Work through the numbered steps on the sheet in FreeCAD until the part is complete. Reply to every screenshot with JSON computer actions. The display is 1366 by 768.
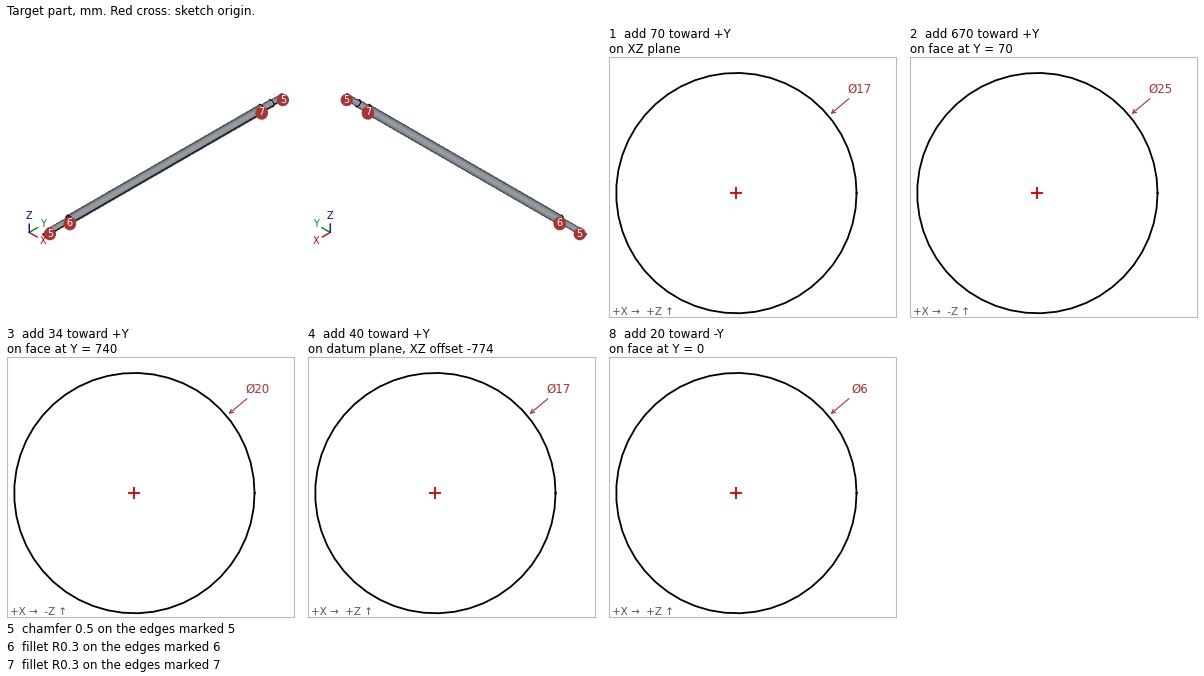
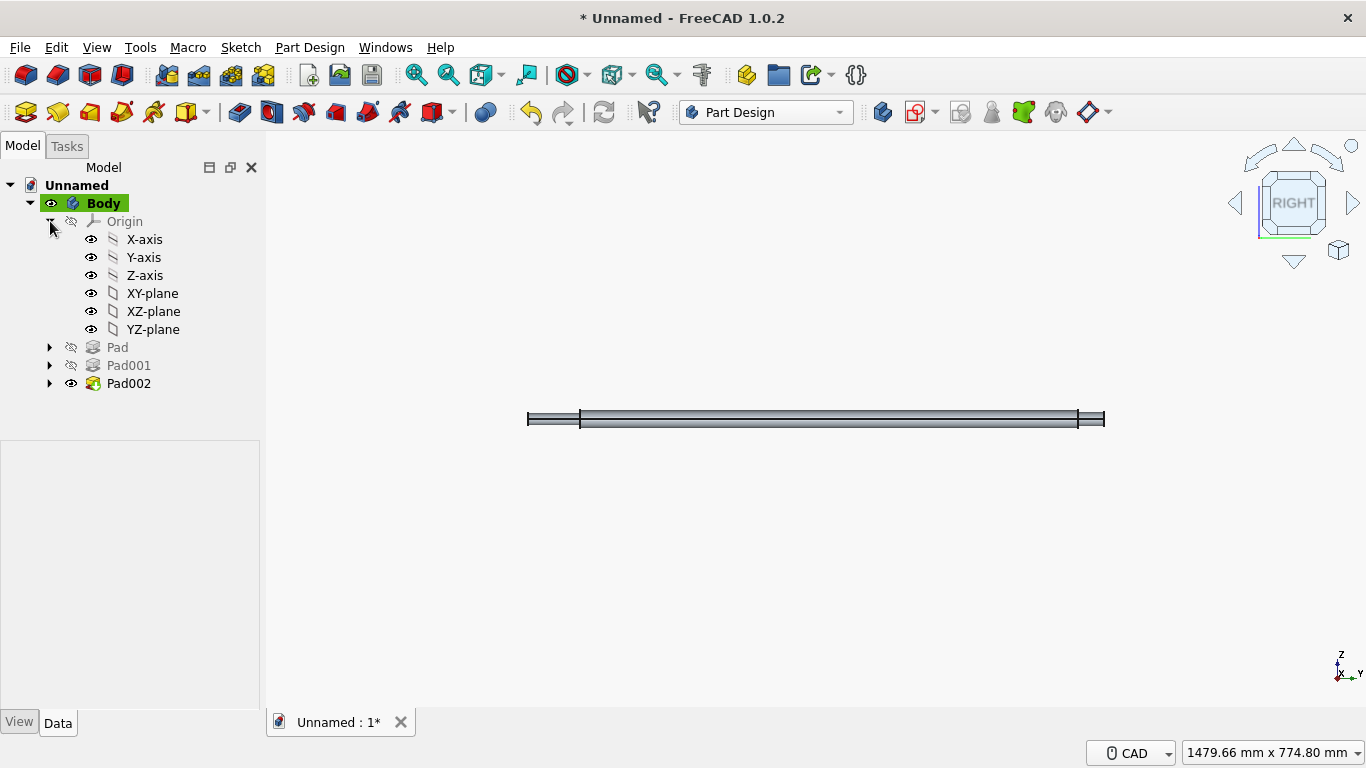
{"action": "left_click", "coordinate": [136, 311]}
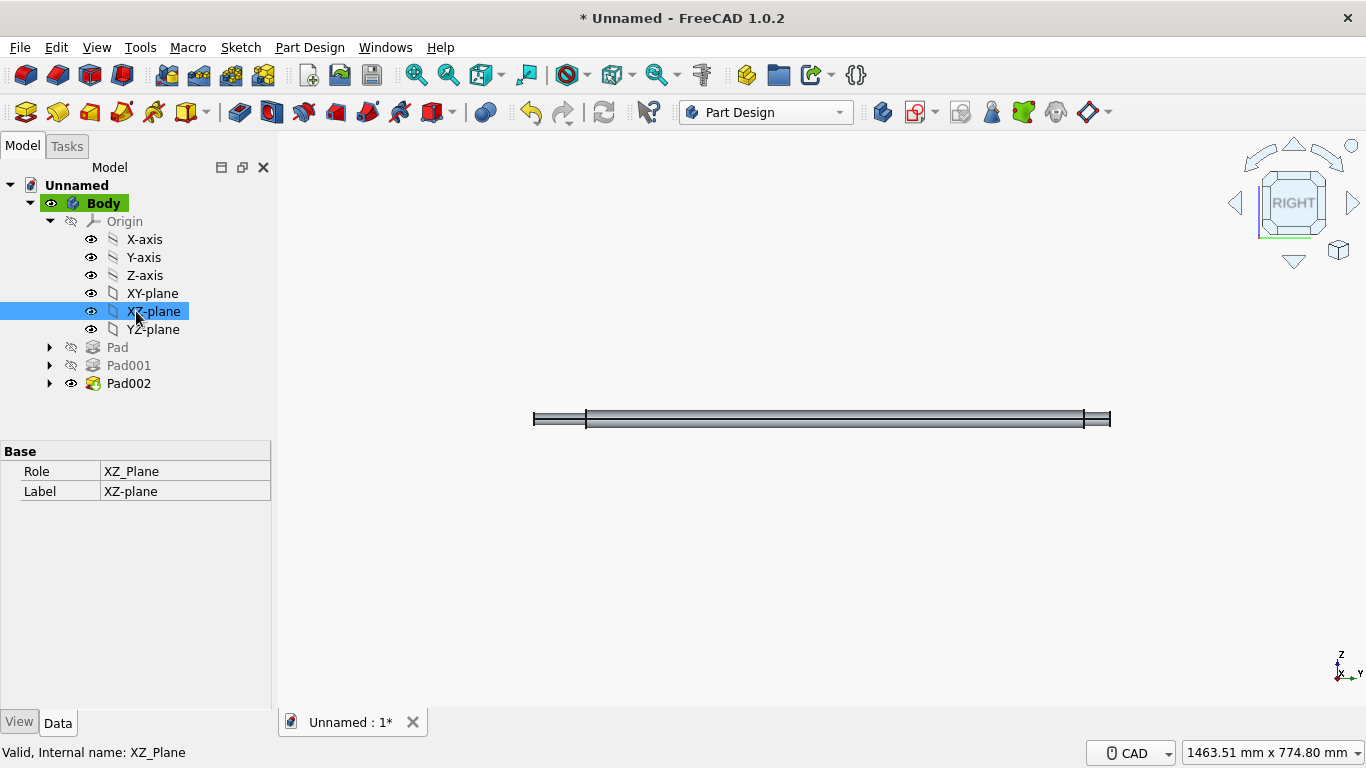
{"action": "left_click", "coordinate": [1088, 112]}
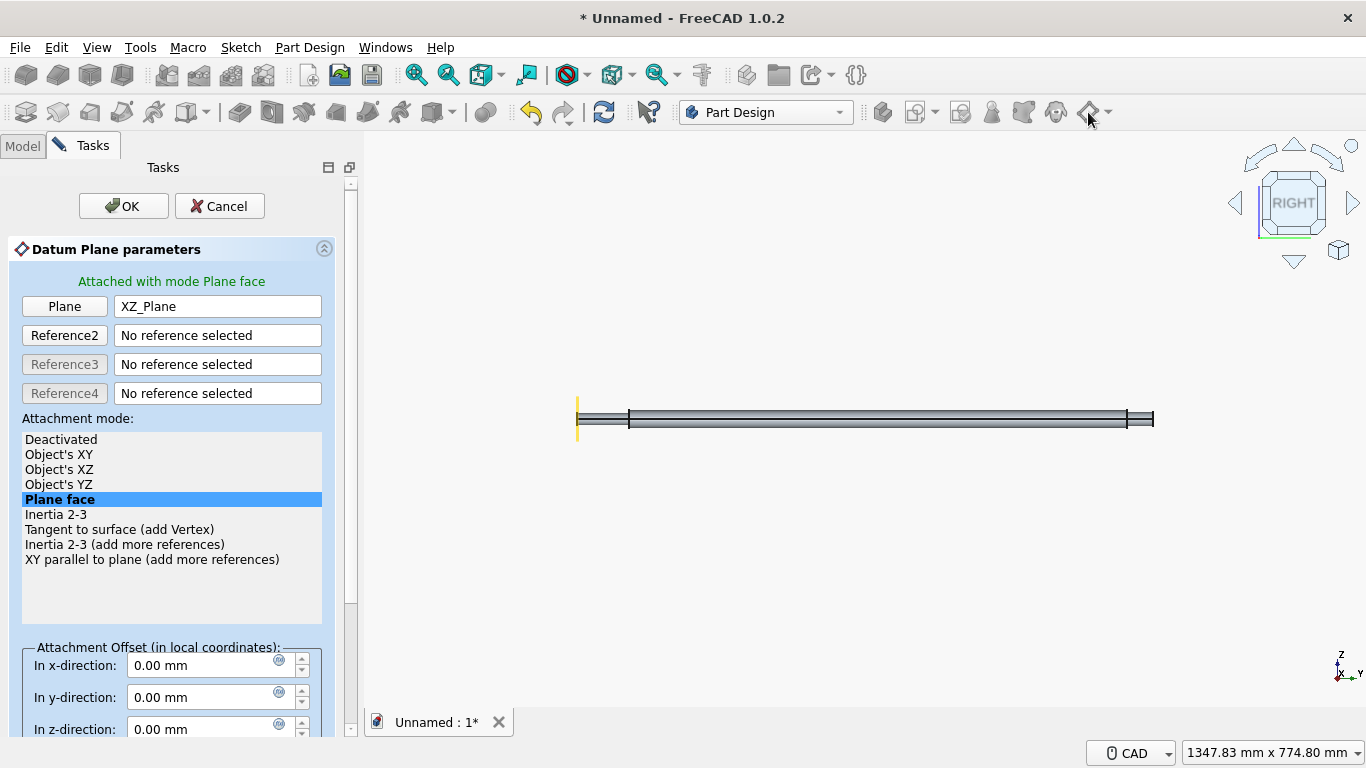
{"action": "scroll", "coordinate": [351, 456], "scroll_direction": "down", "scroll_amount": 2}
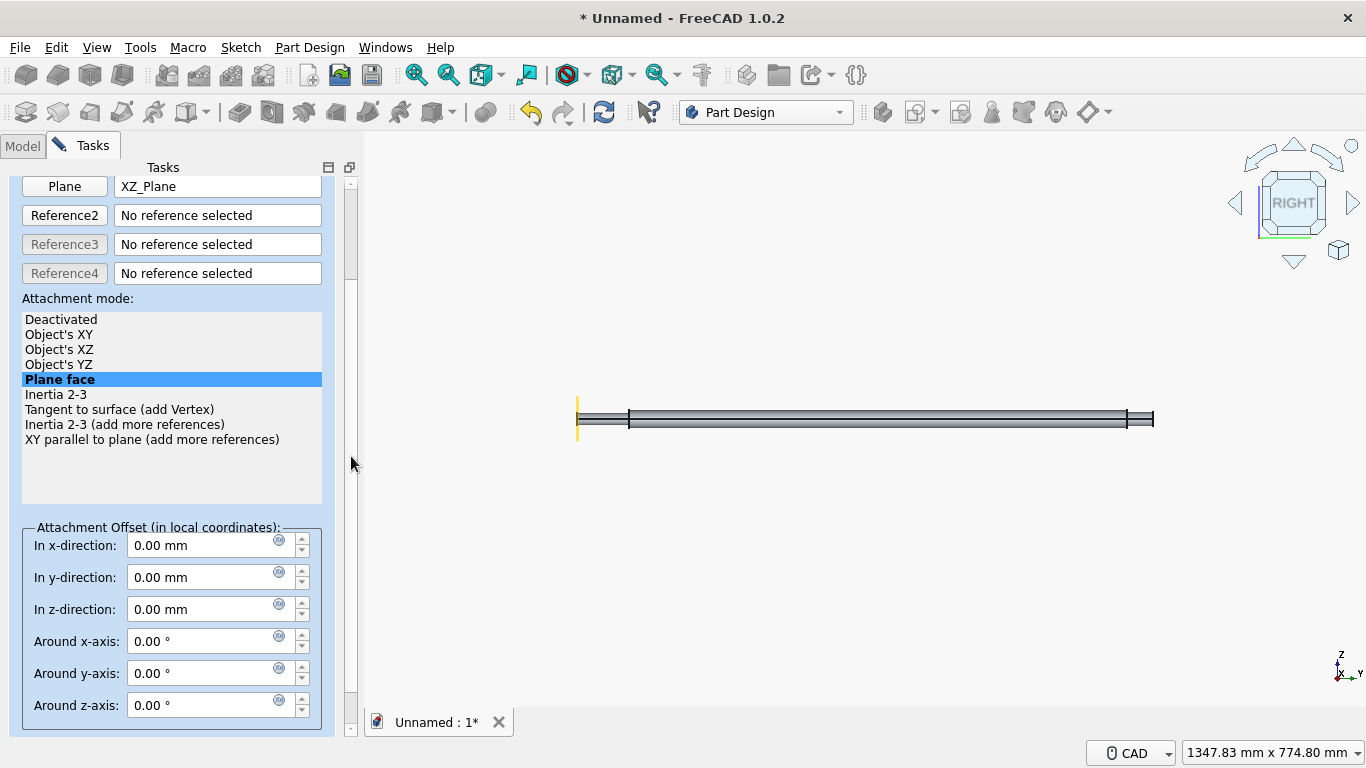
{"action": "triple_click", "coordinate": [210, 609]}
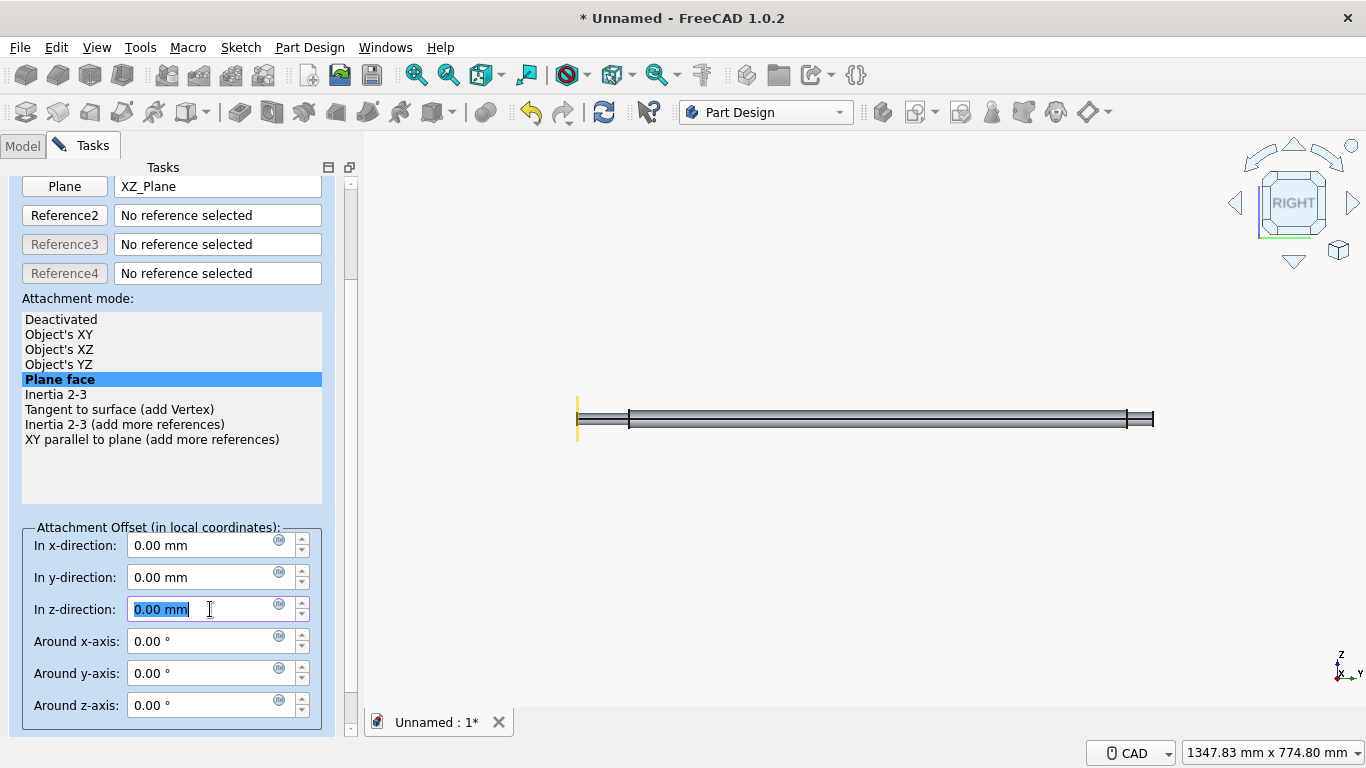
{"action": "type", "text": "-774"}
{"action": "key", "text": "Tab"}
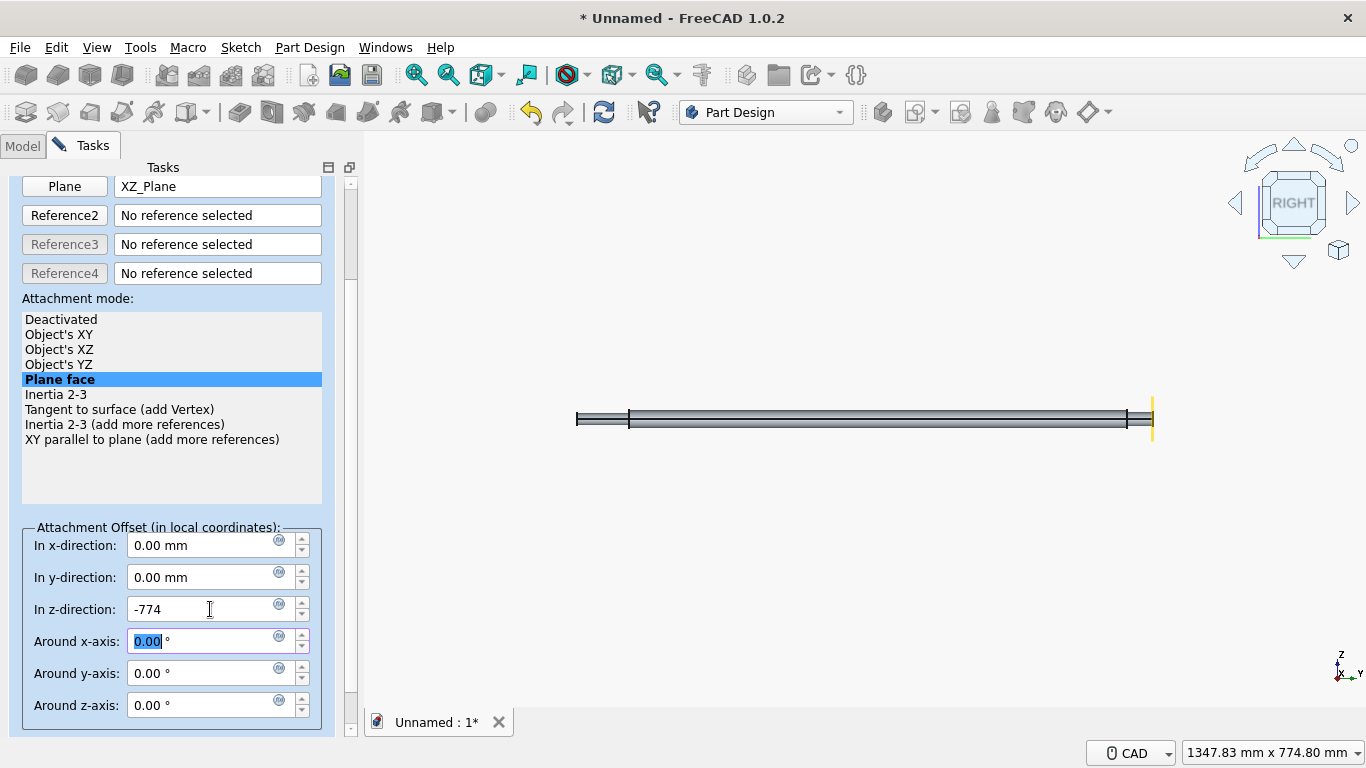
{"action": "scroll", "coordinate": [351, 456], "scroll_direction": "up", "scroll_amount": 3}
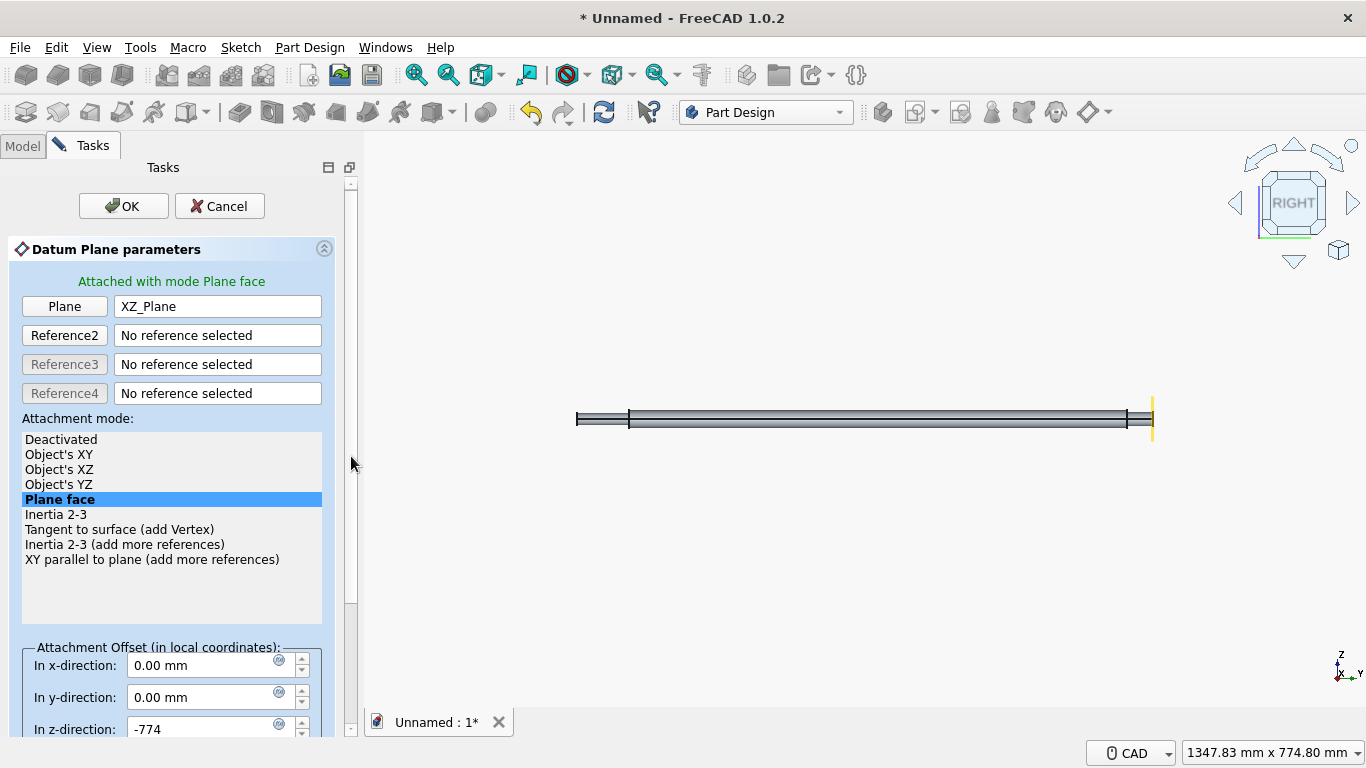
{"action": "left_click", "coordinate": [124, 206]}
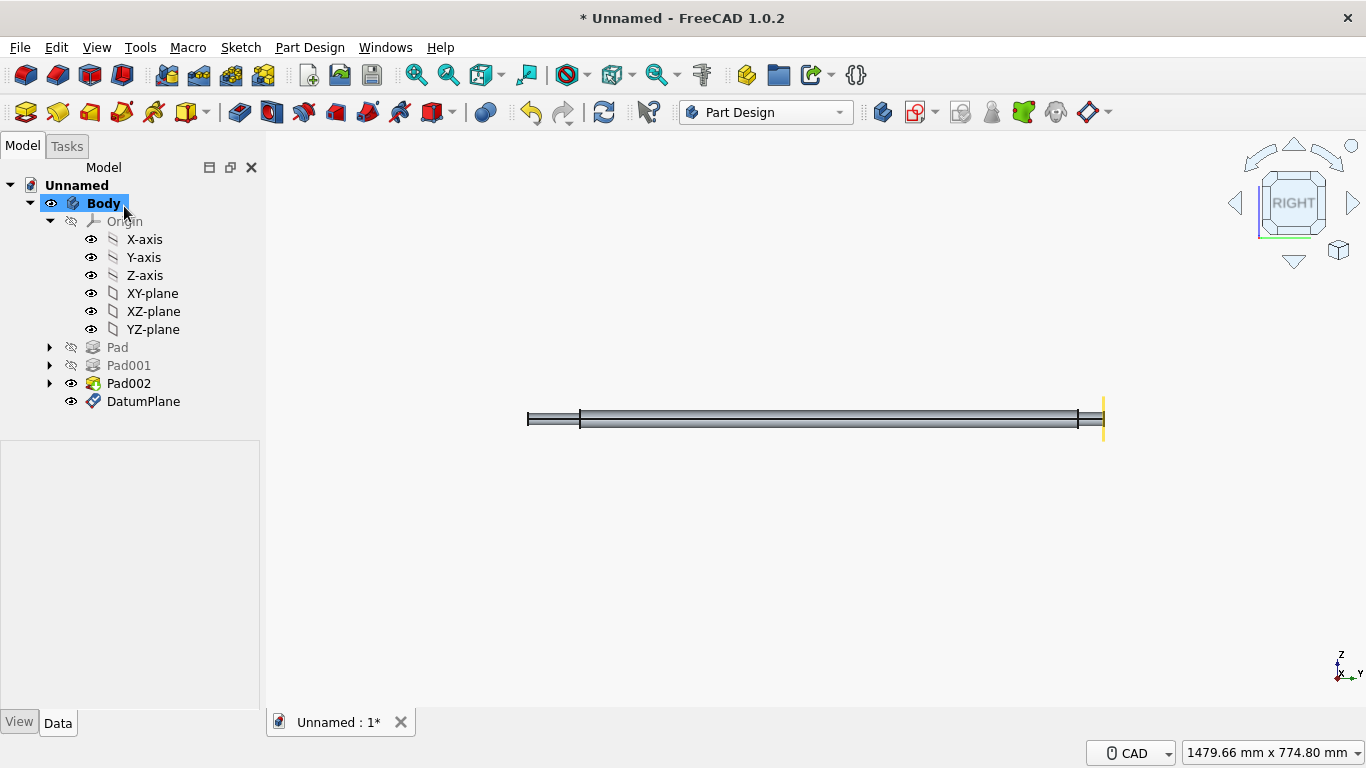
{"action": "left_click", "coordinate": [116, 401]}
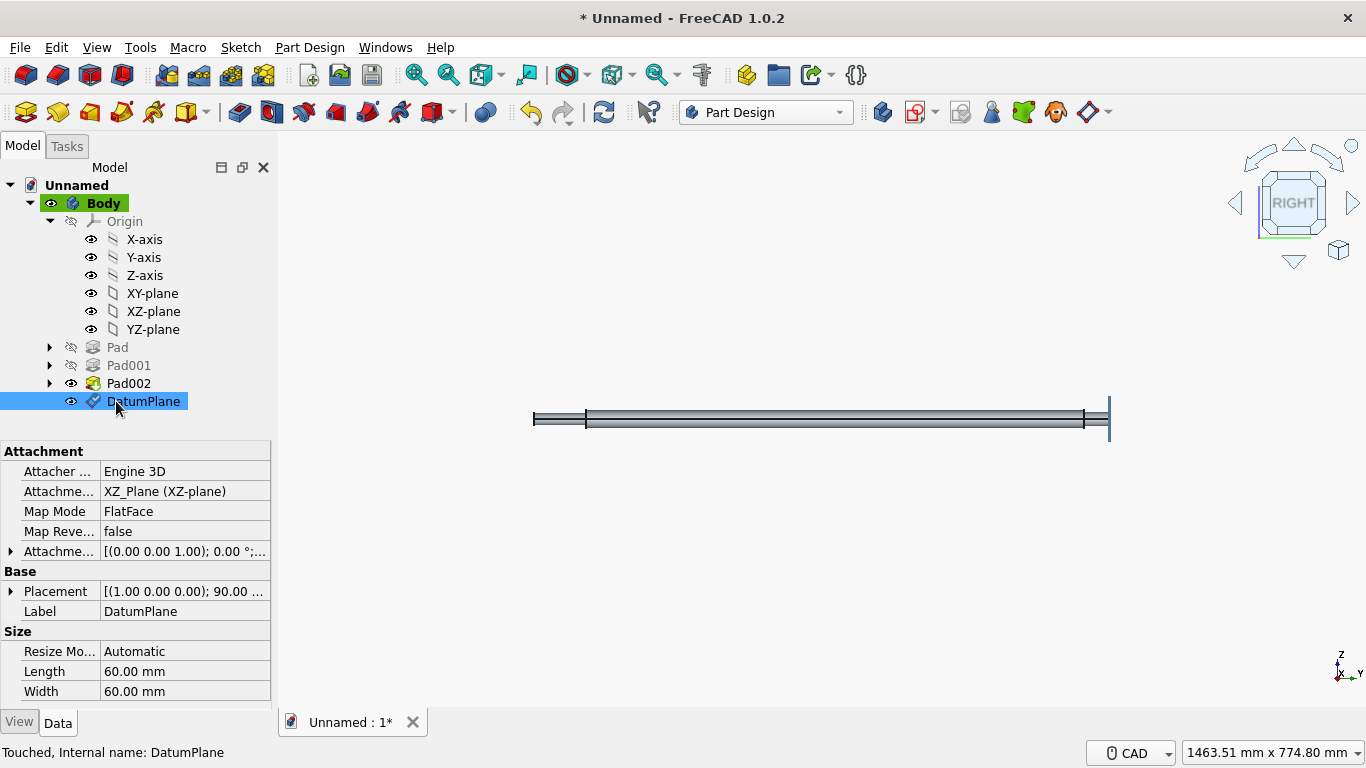
{"action": "left_click", "coordinate": [916, 112]}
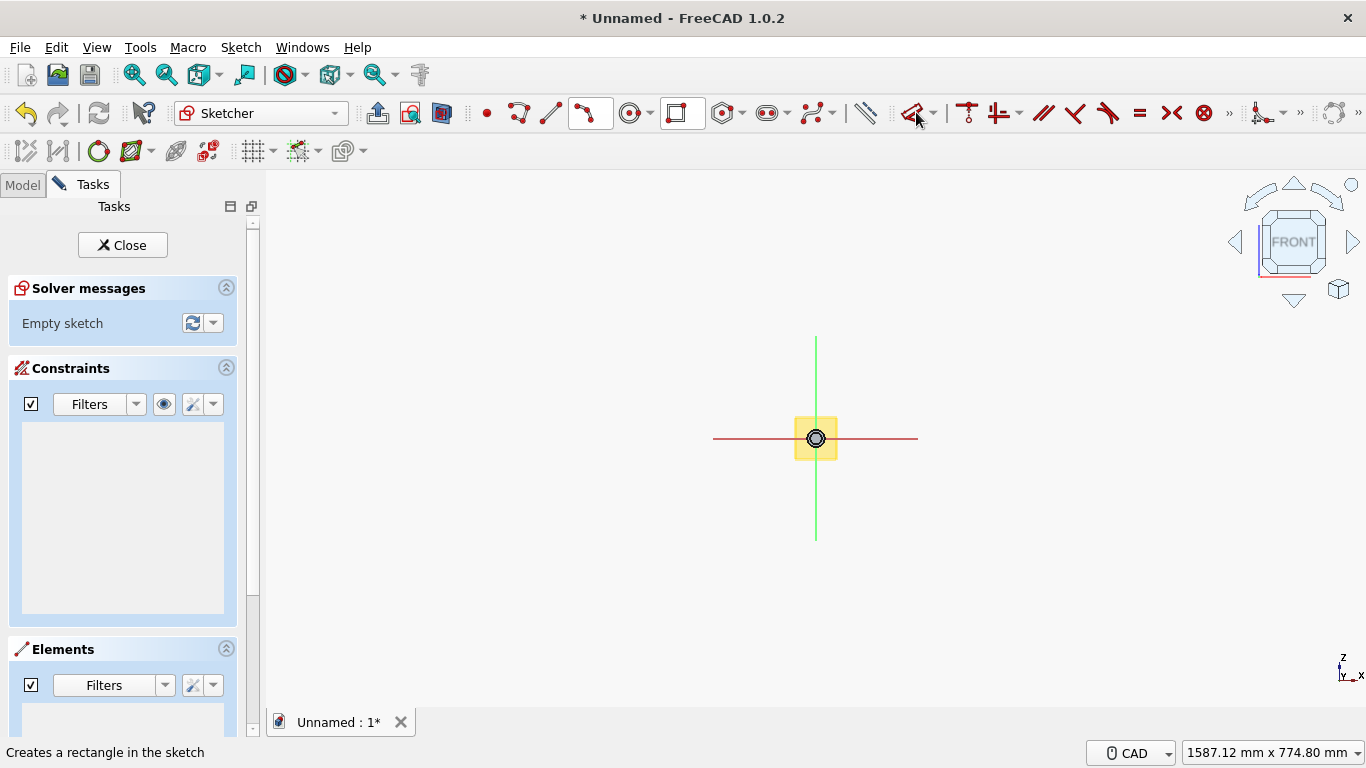
{"action": "left_click", "coordinate": [442, 114]}